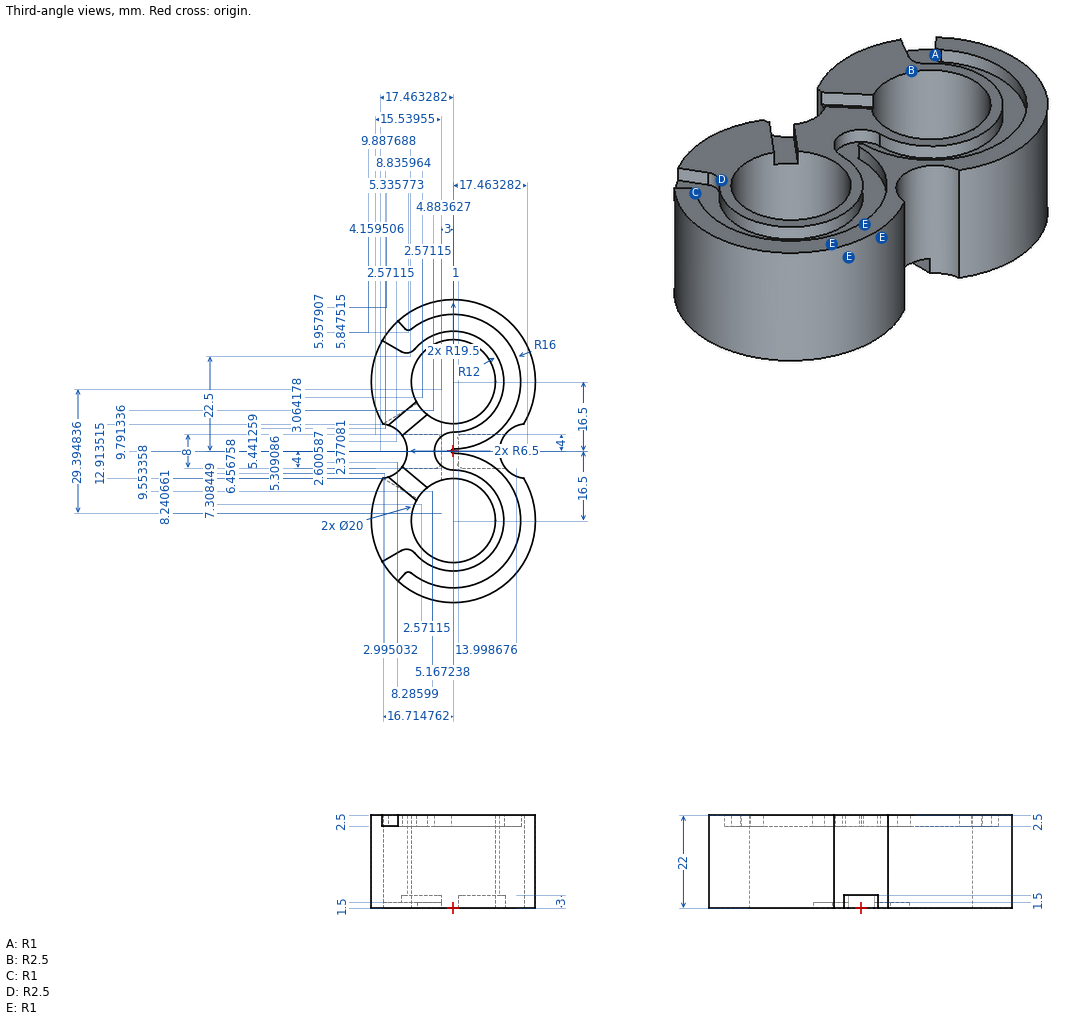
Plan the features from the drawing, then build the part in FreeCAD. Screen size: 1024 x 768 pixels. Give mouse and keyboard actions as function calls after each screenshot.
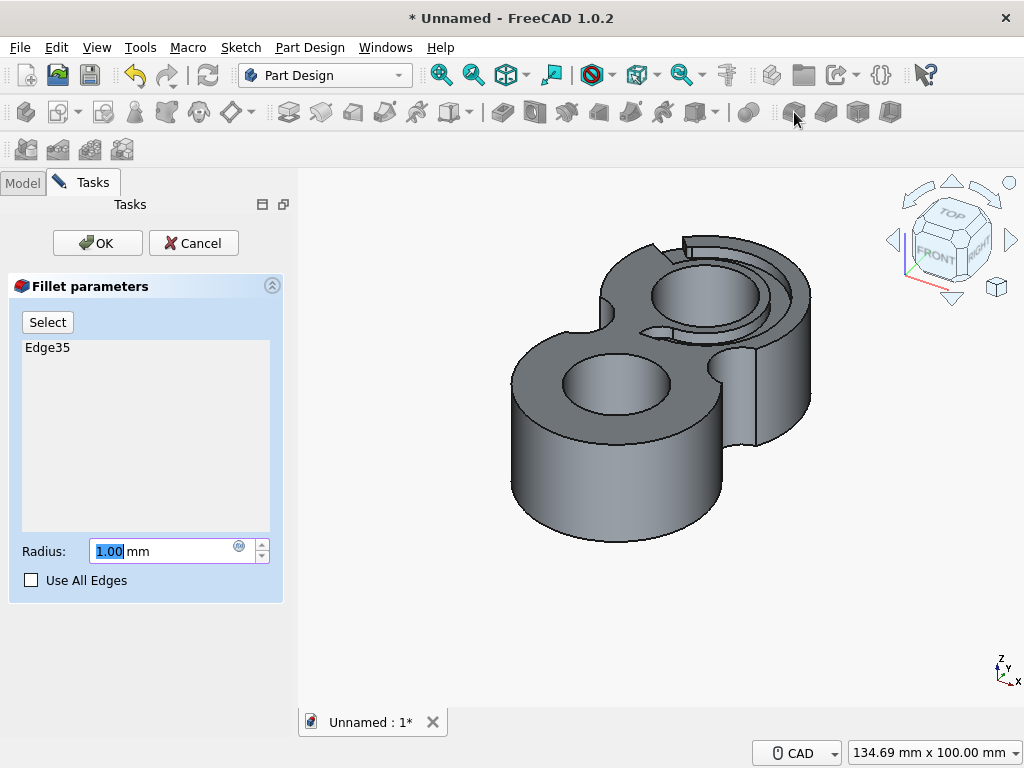
text(1)
key(Tab)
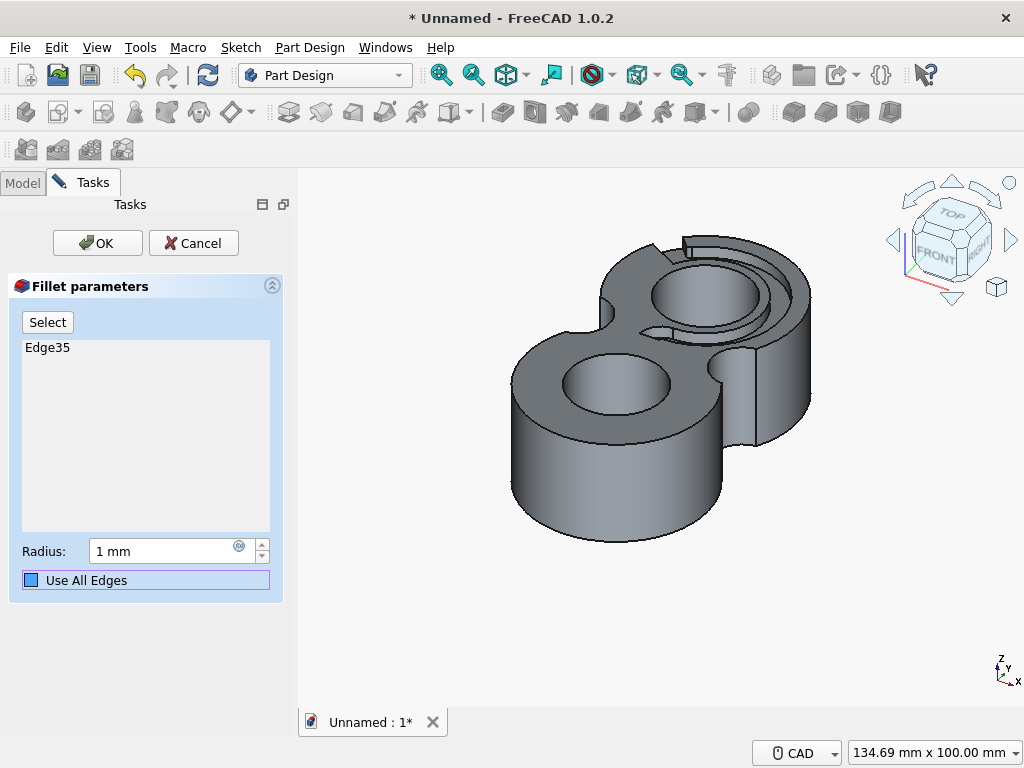
click(98, 243)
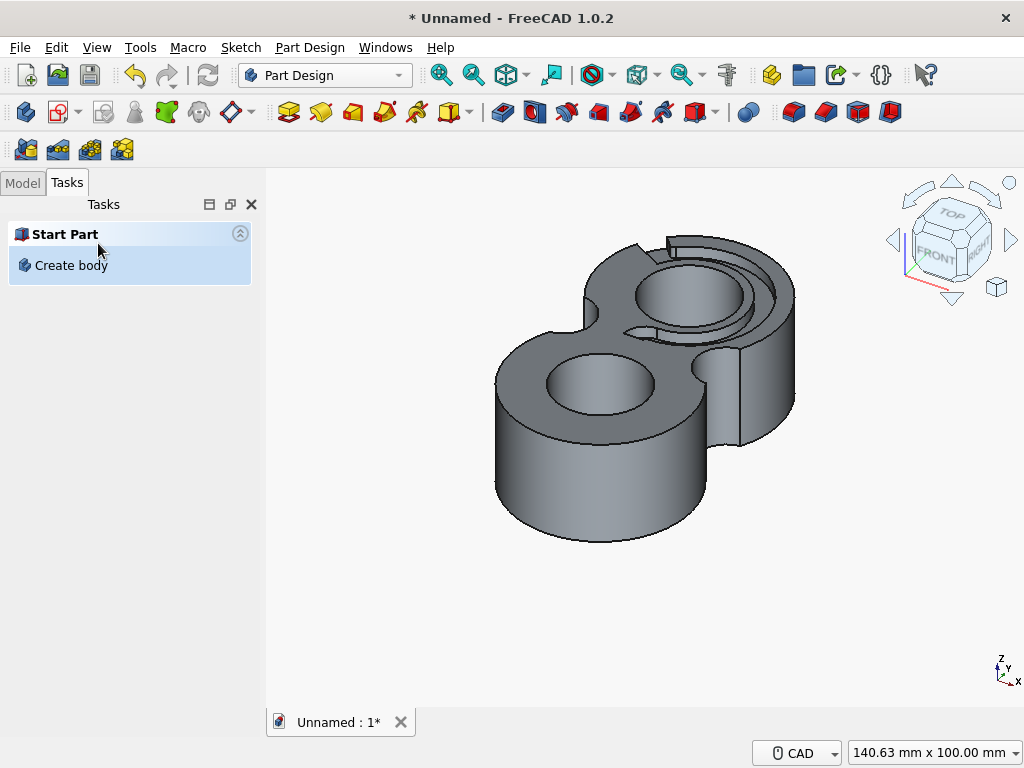
scroll(657, 269, up, 6)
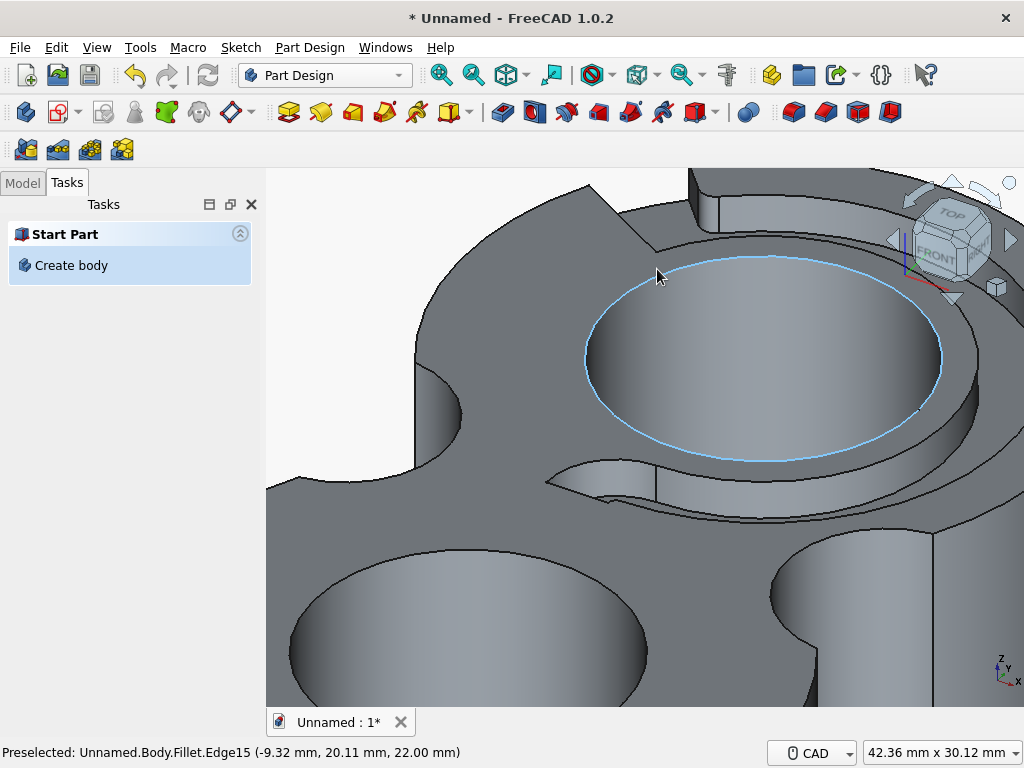
key(v)
key(f)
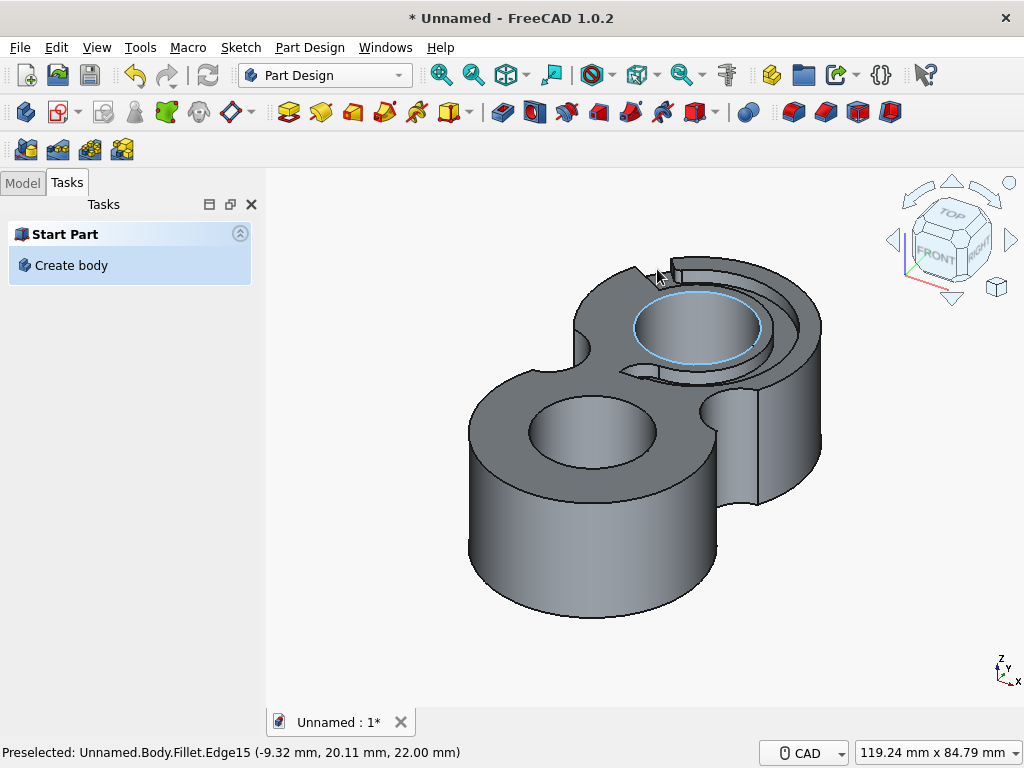
key(0)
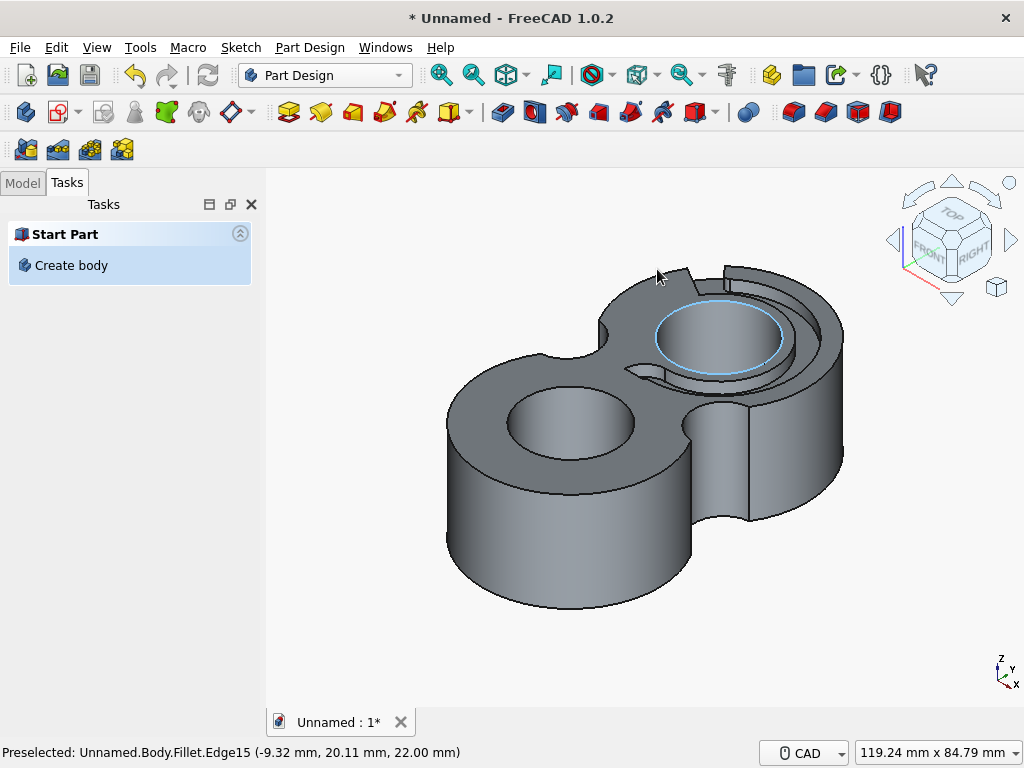
scroll(699, 301, up, 5)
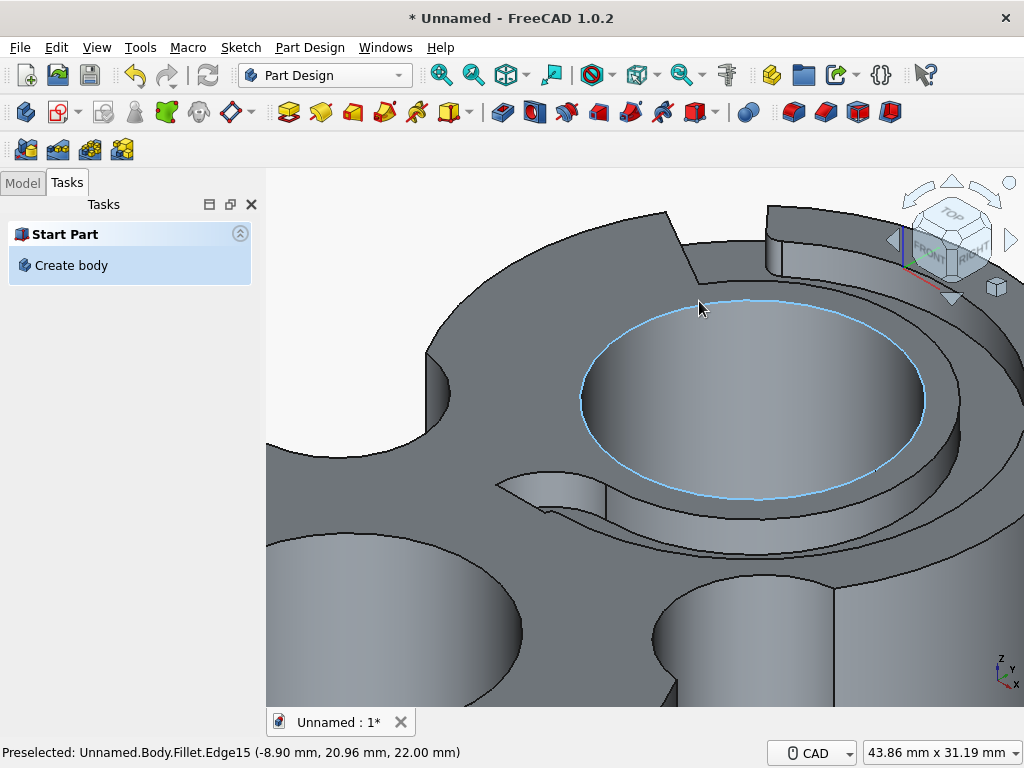
key(v)
key(f)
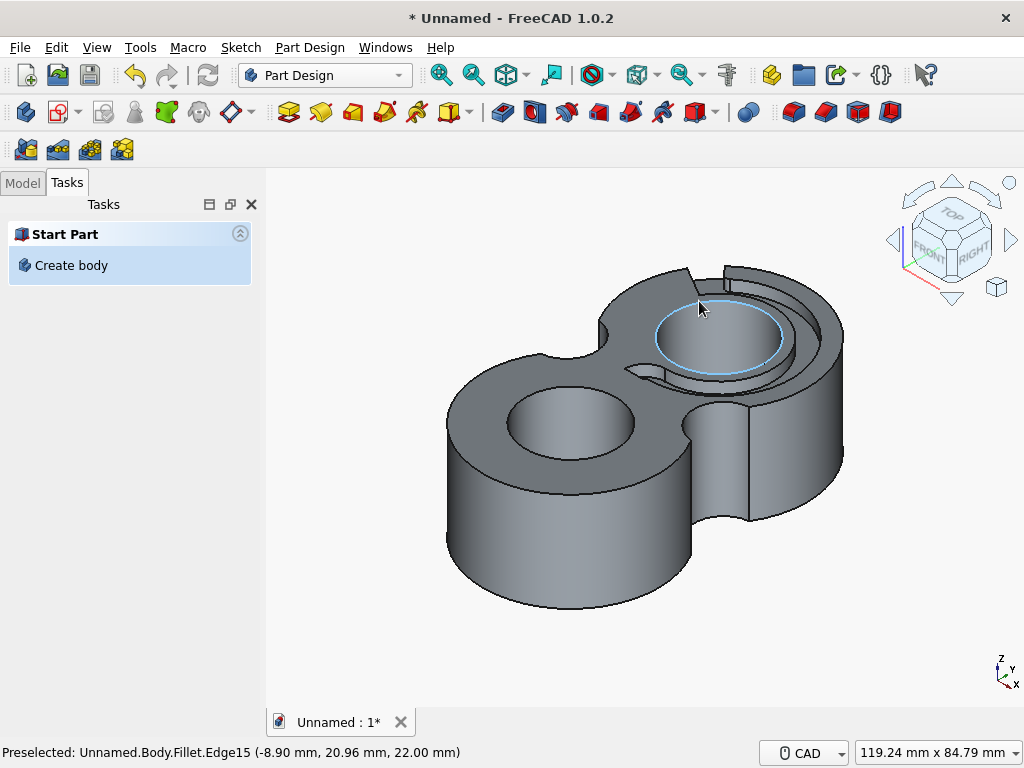
key(2)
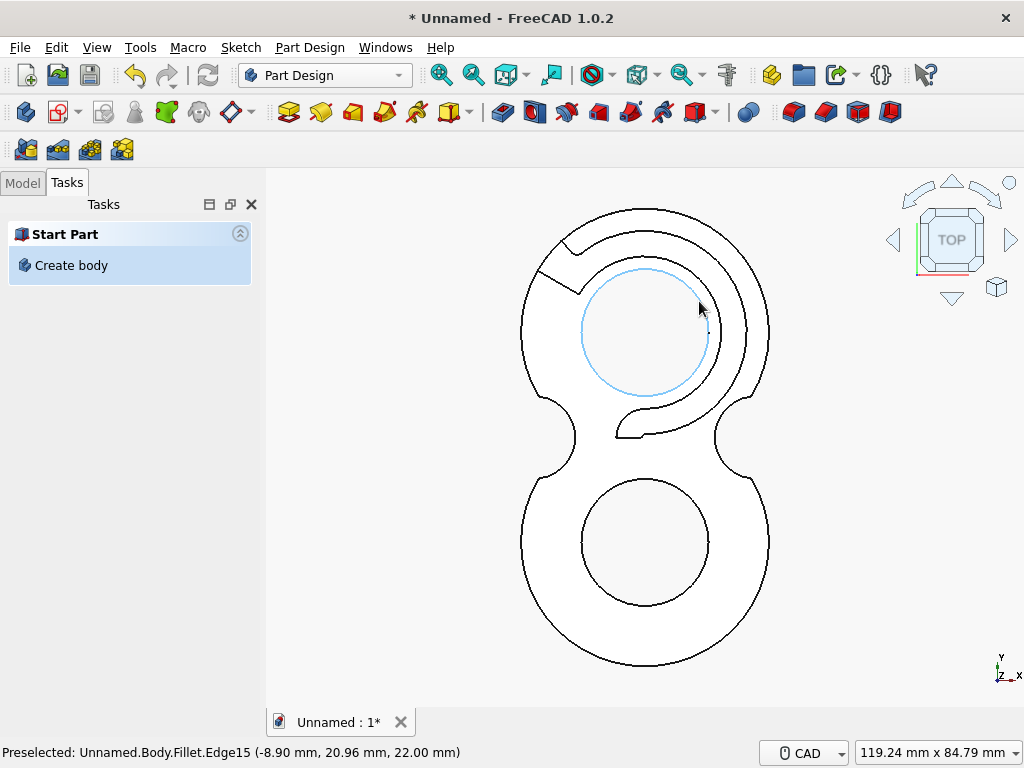
scroll(579, 293, up, 5)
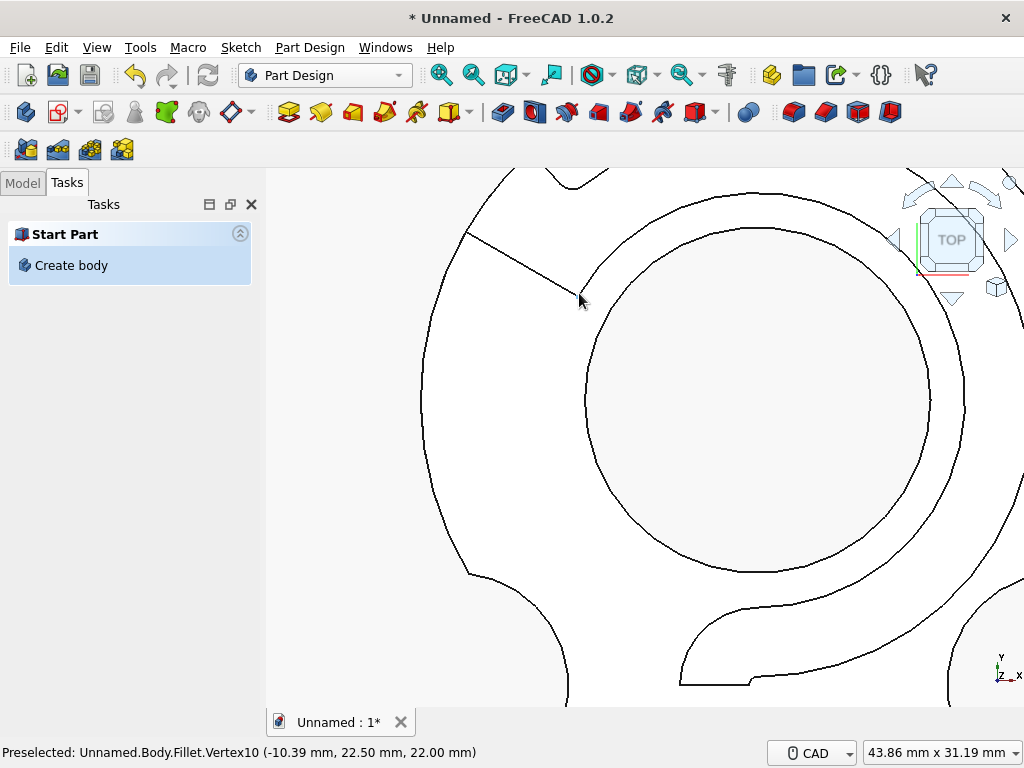
key(v)
key(f)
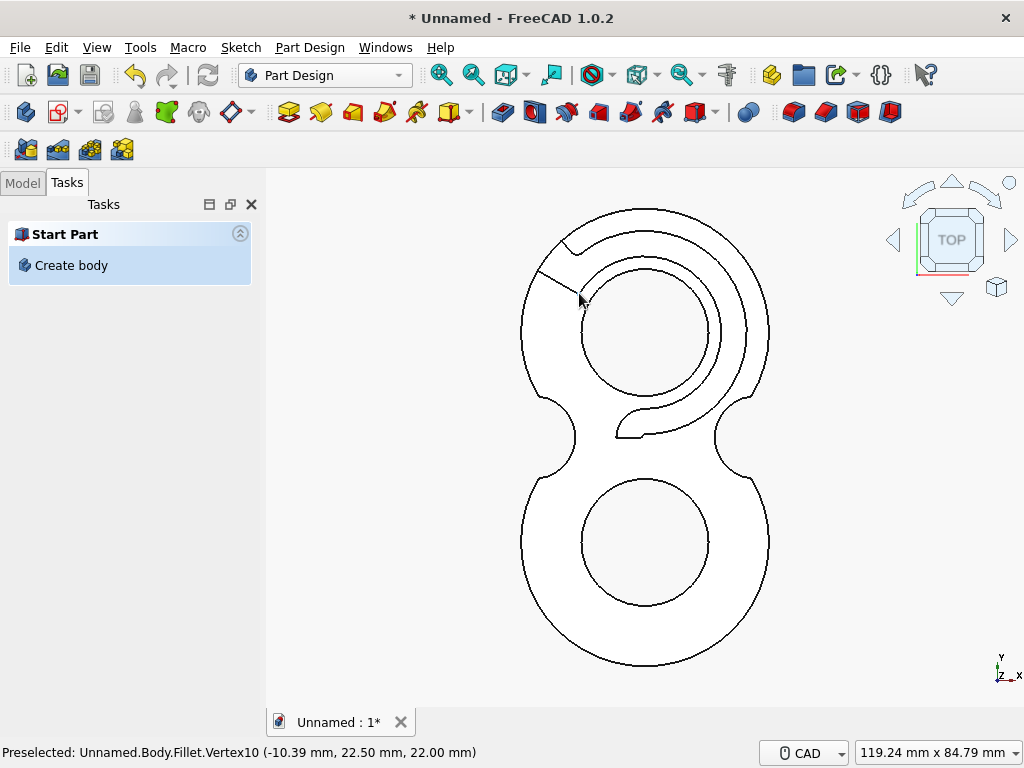
key(1)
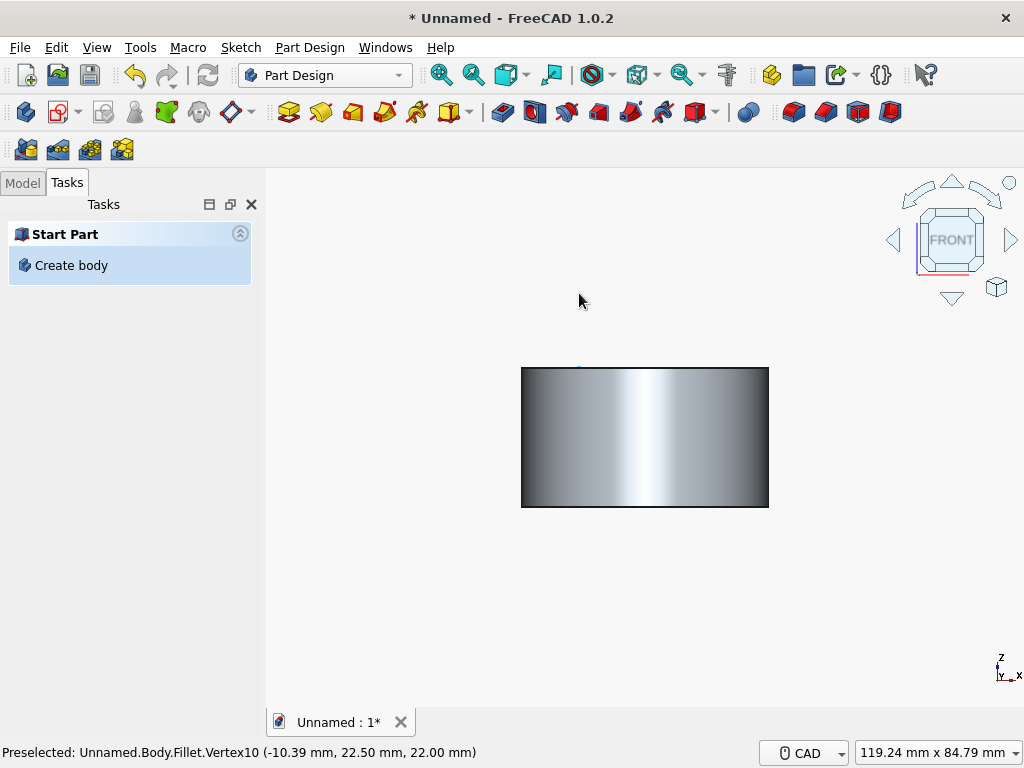
key(v)
key(f)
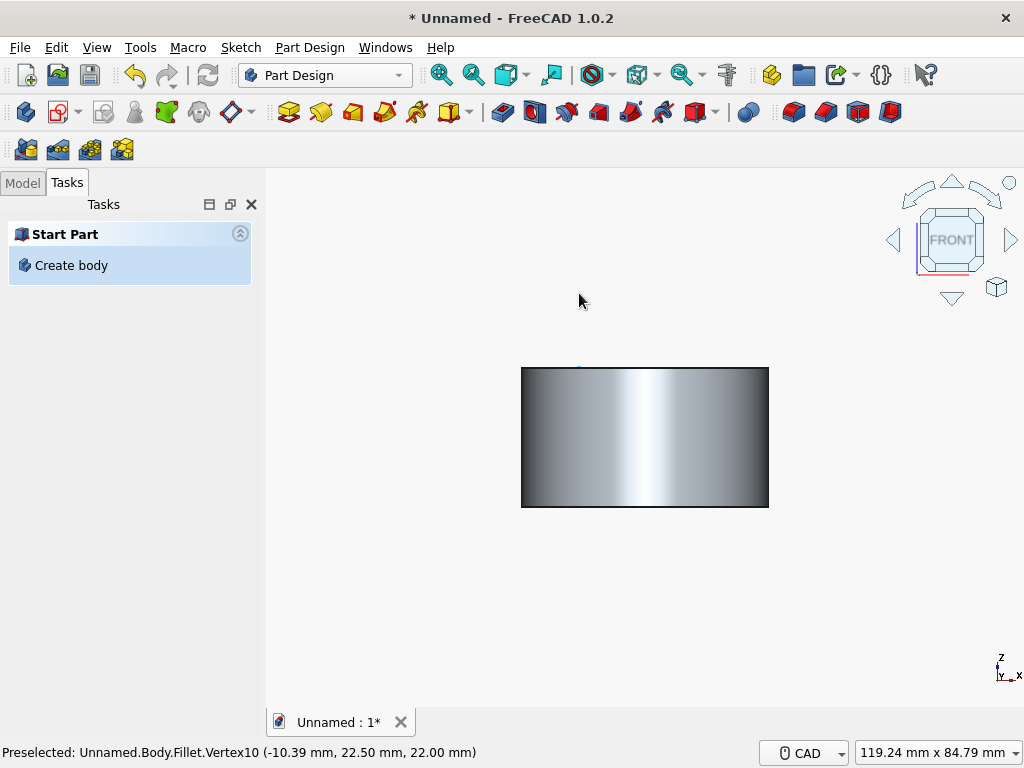
scroll(579, 375, up, 5)